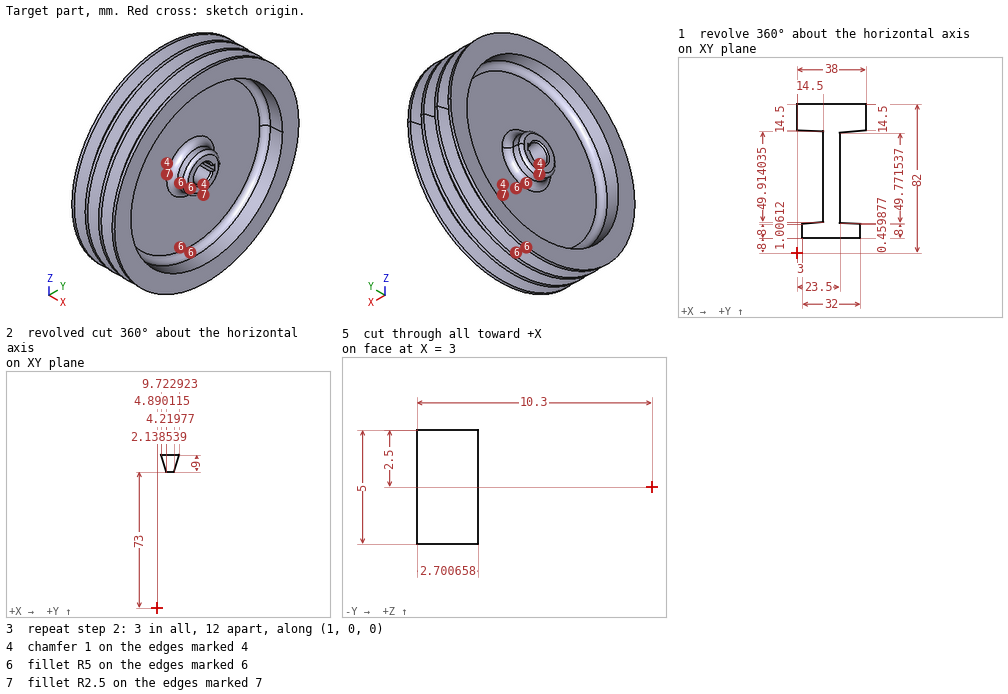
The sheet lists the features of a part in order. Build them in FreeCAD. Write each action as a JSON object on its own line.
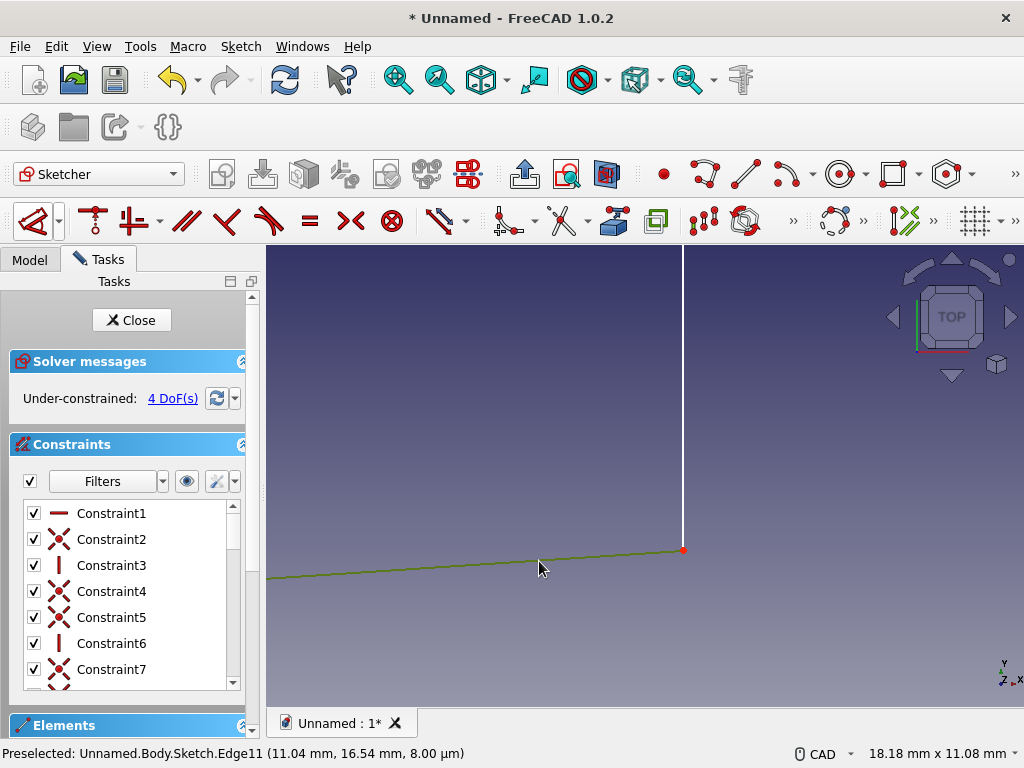
{"action": "left_click", "coordinate": [58, 222]}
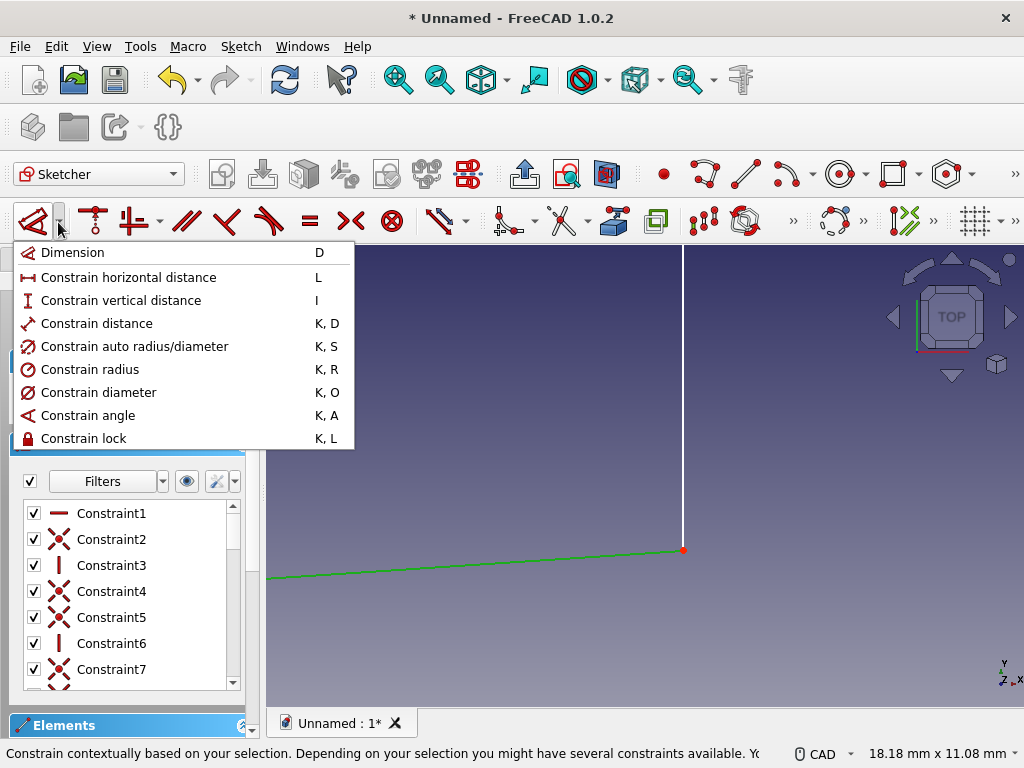
{"action": "left_click", "coordinate": [184, 300]}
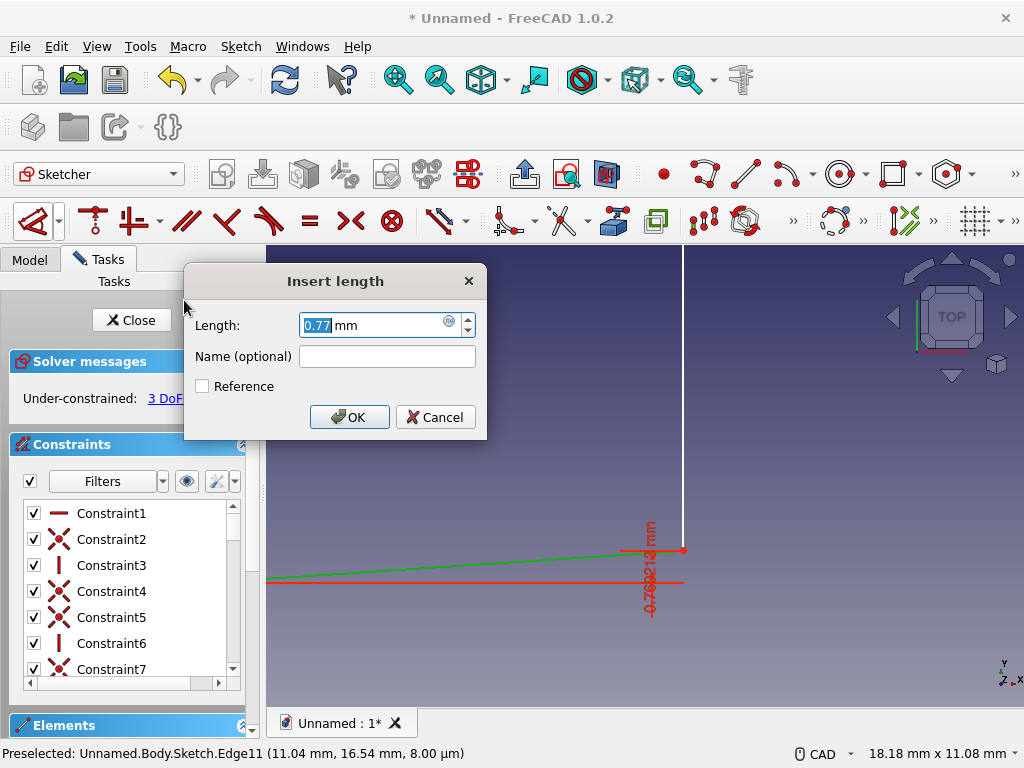
{"action": "type", "text": "1.00612"}
{"action": "key", "text": "Return"}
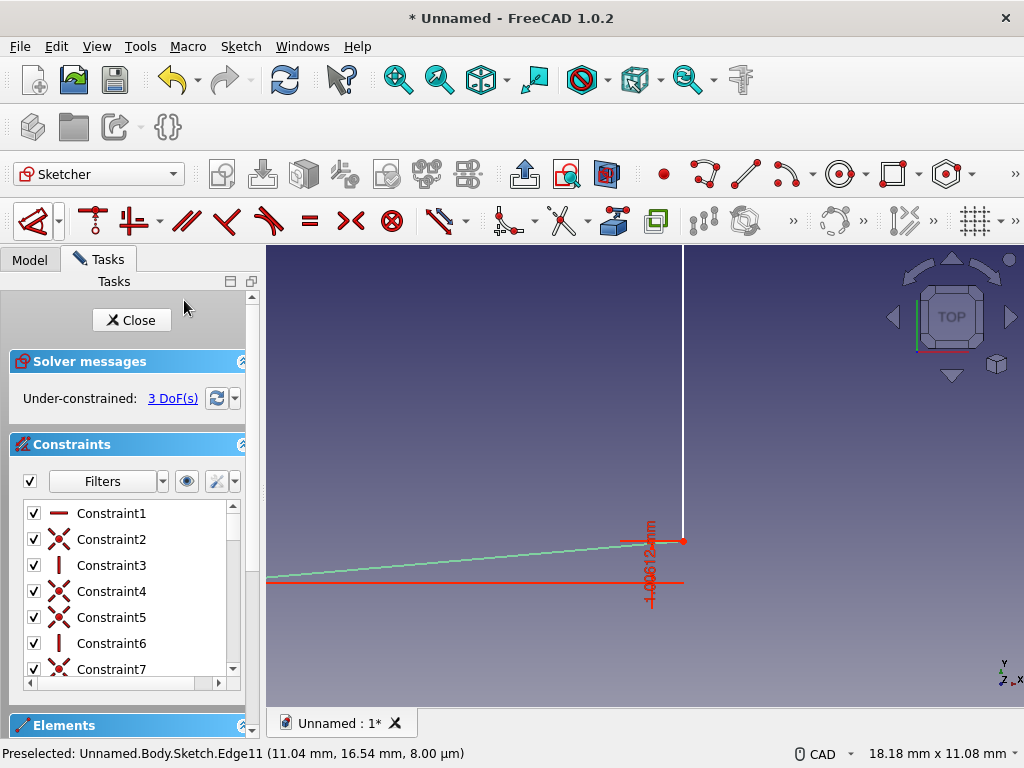
{"action": "scroll", "coordinate": [547, 569], "scroll_direction": "down", "scroll_amount": 12}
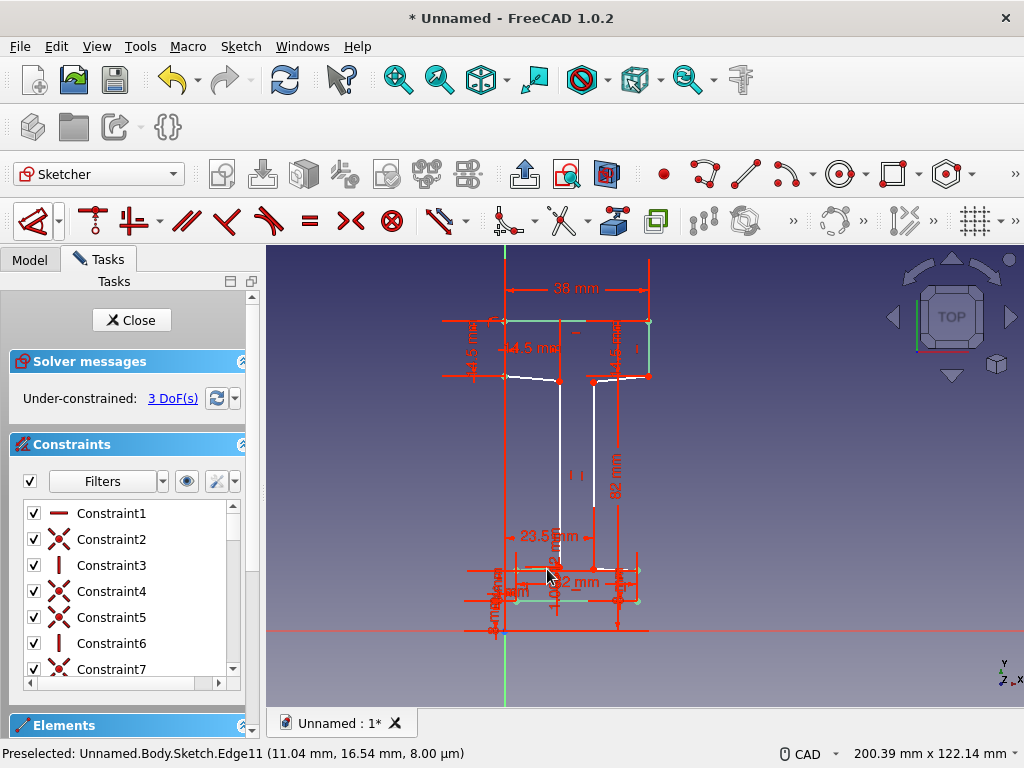
{"action": "left_click", "coordinate": [594, 513]}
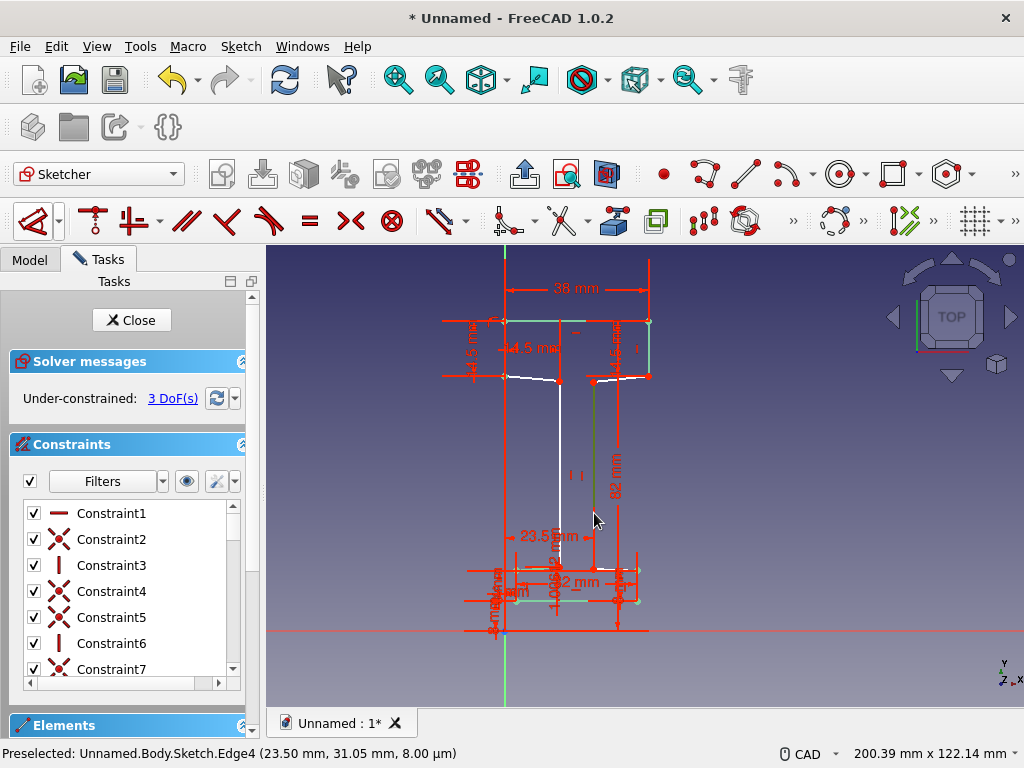
{"action": "left_click", "coordinate": [58, 222]}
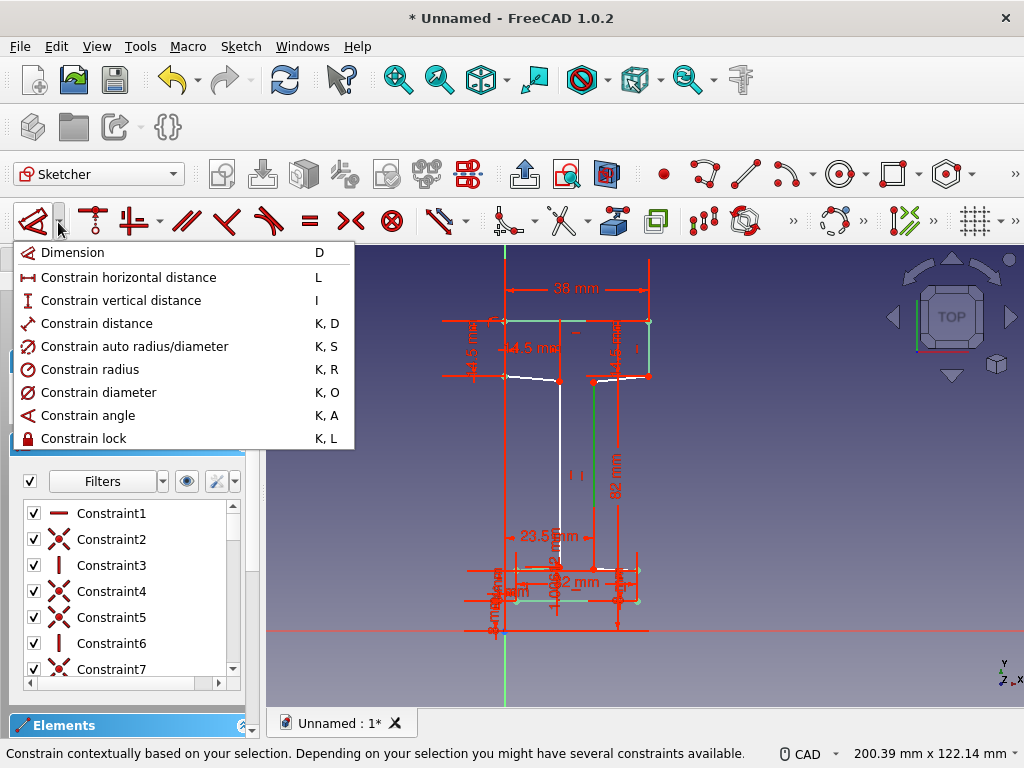
{"action": "left_click", "coordinate": [184, 300]}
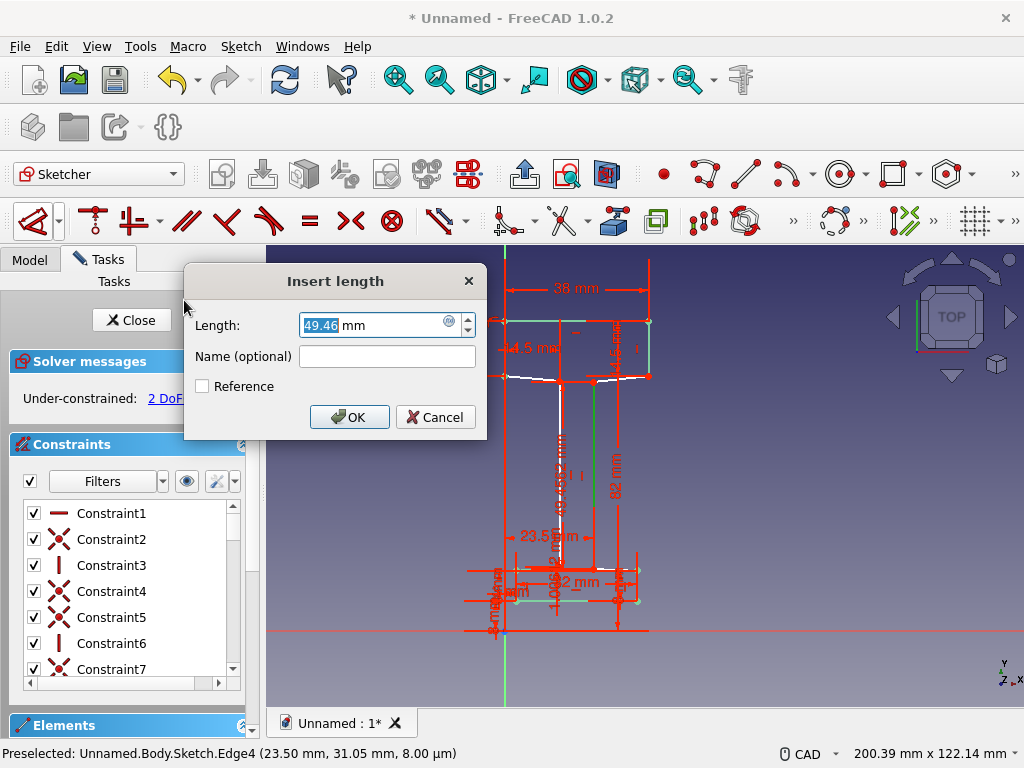
{"action": "type", "text": "49.771537"}
{"action": "key", "text": "Return"}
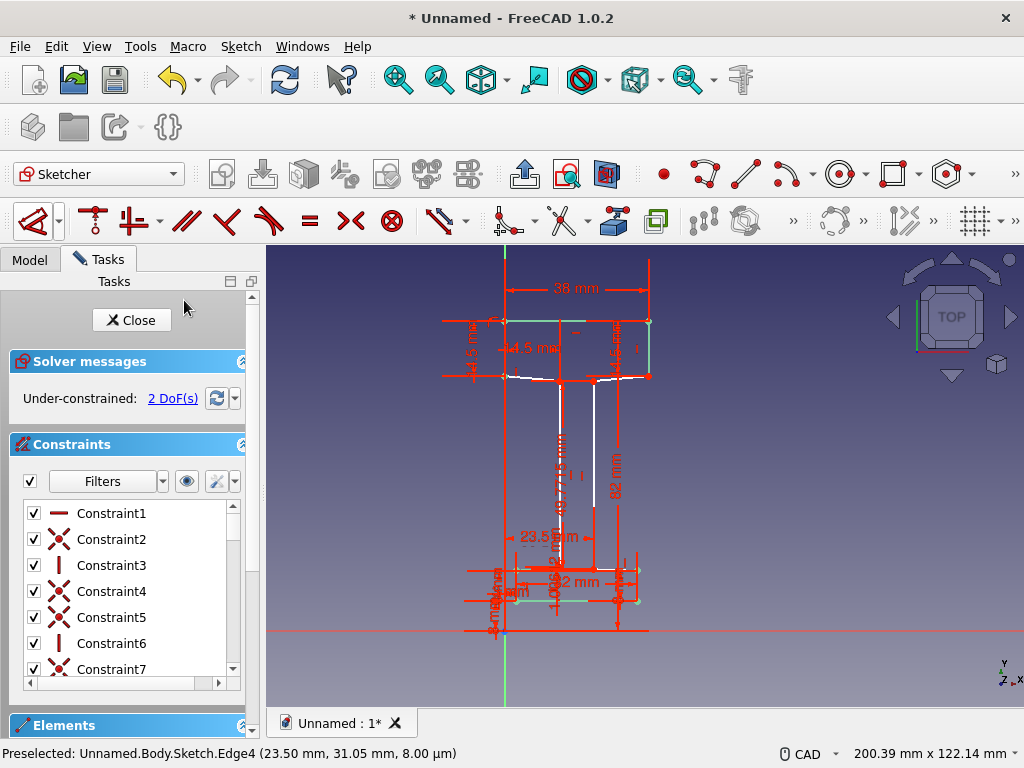
{"action": "left_click", "coordinate": [560, 418]}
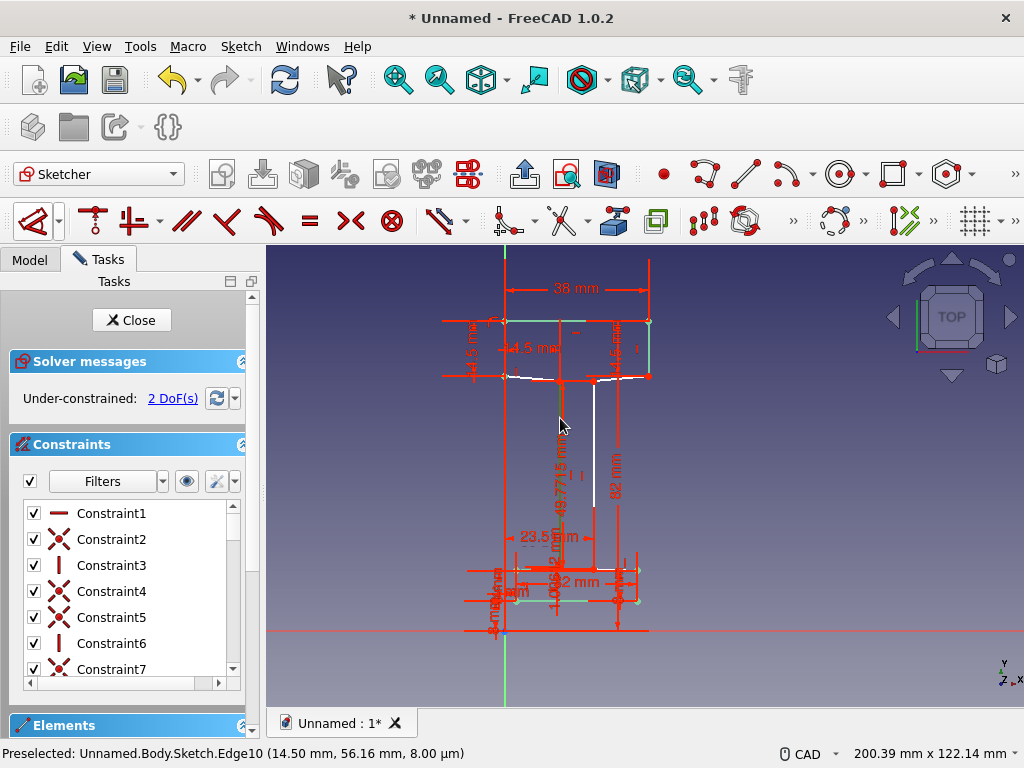
{"action": "key", "text": "i"}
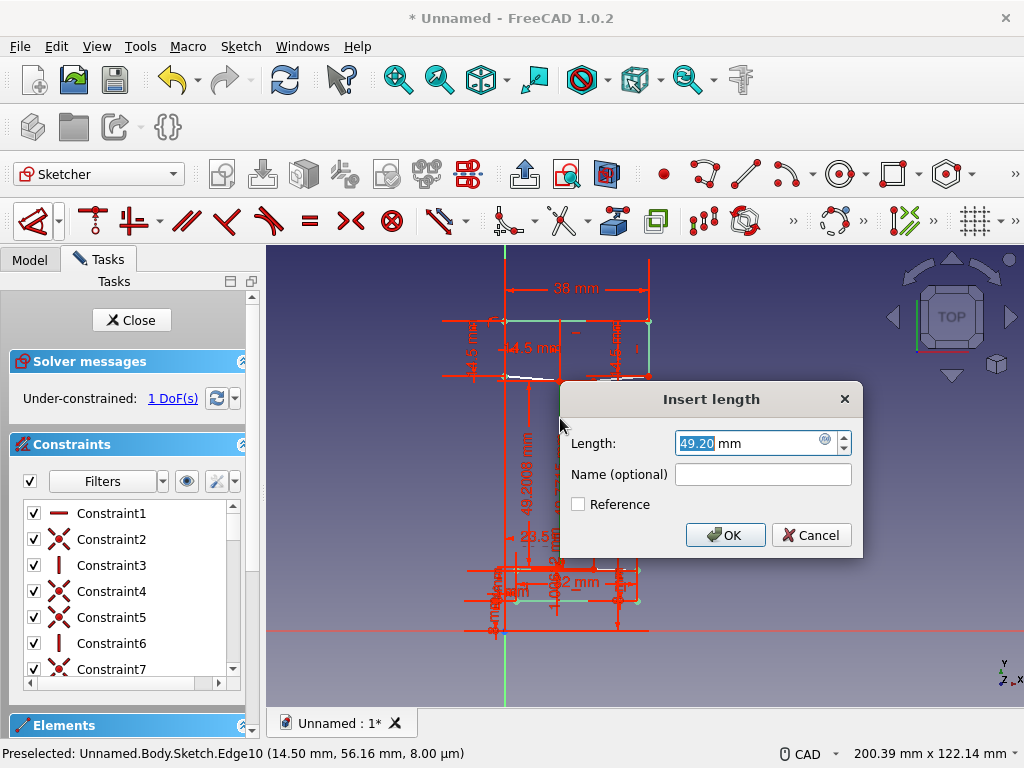
{"action": "type", "text": "49.914035"}
{"action": "key", "text": "Return"}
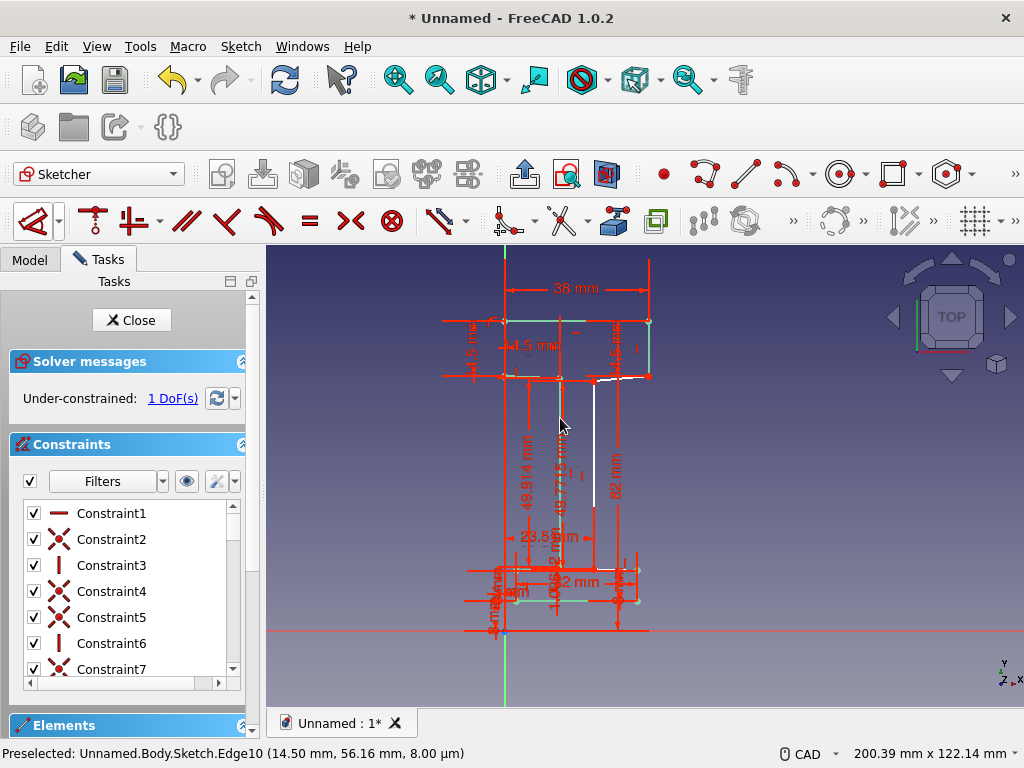
{"action": "scroll", "coordinate": [624, 570], "scroll_direction": "up", "scroll_amount": 16}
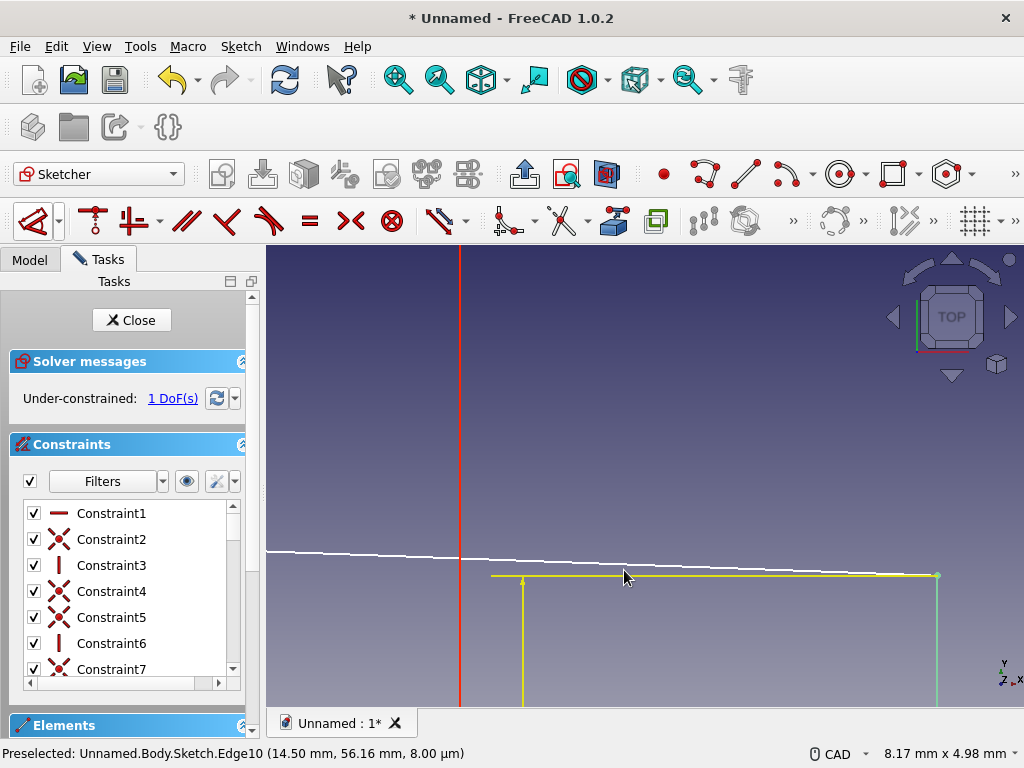
{"action": "left_click", "coordinate": [617, 564]}